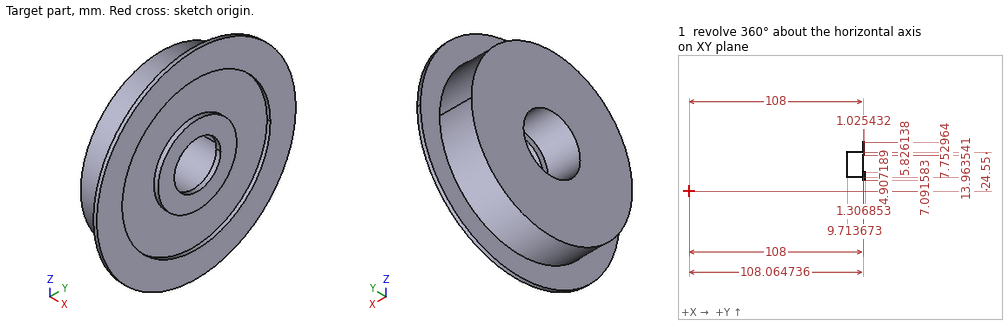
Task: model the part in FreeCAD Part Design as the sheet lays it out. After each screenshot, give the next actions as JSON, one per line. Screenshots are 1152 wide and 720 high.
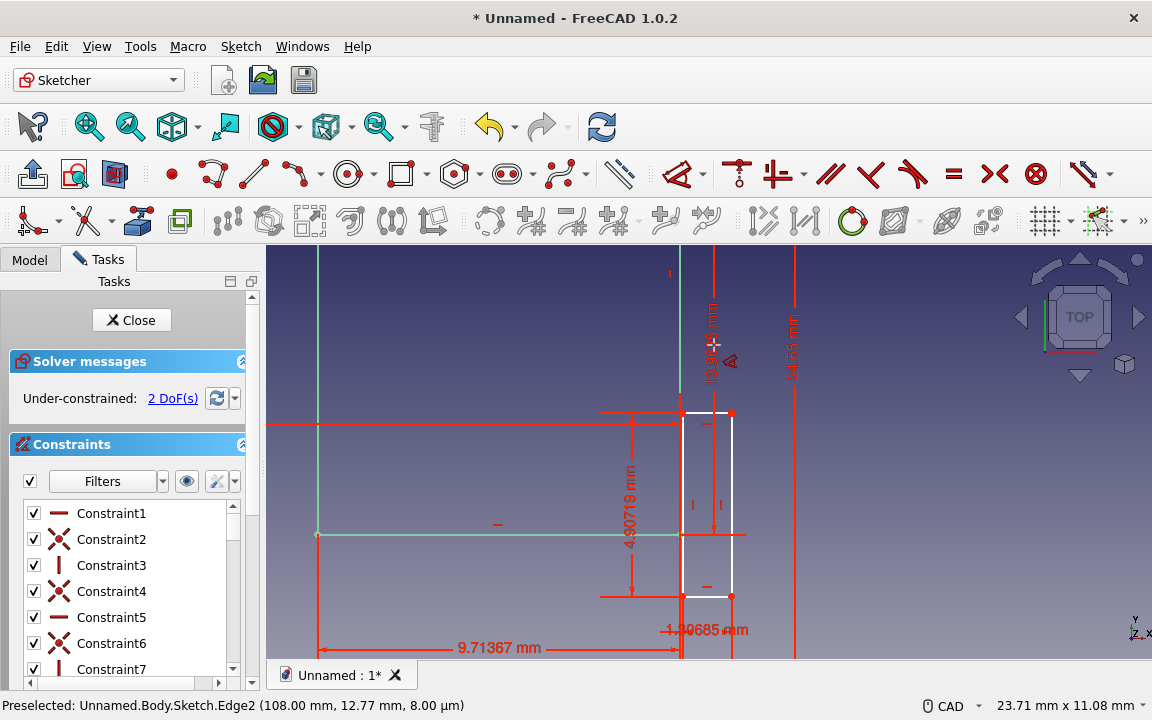
{"action": "left_click", "coordinate": [683, 597]}
{"action": "left_click", "coordinate": [741, 606]}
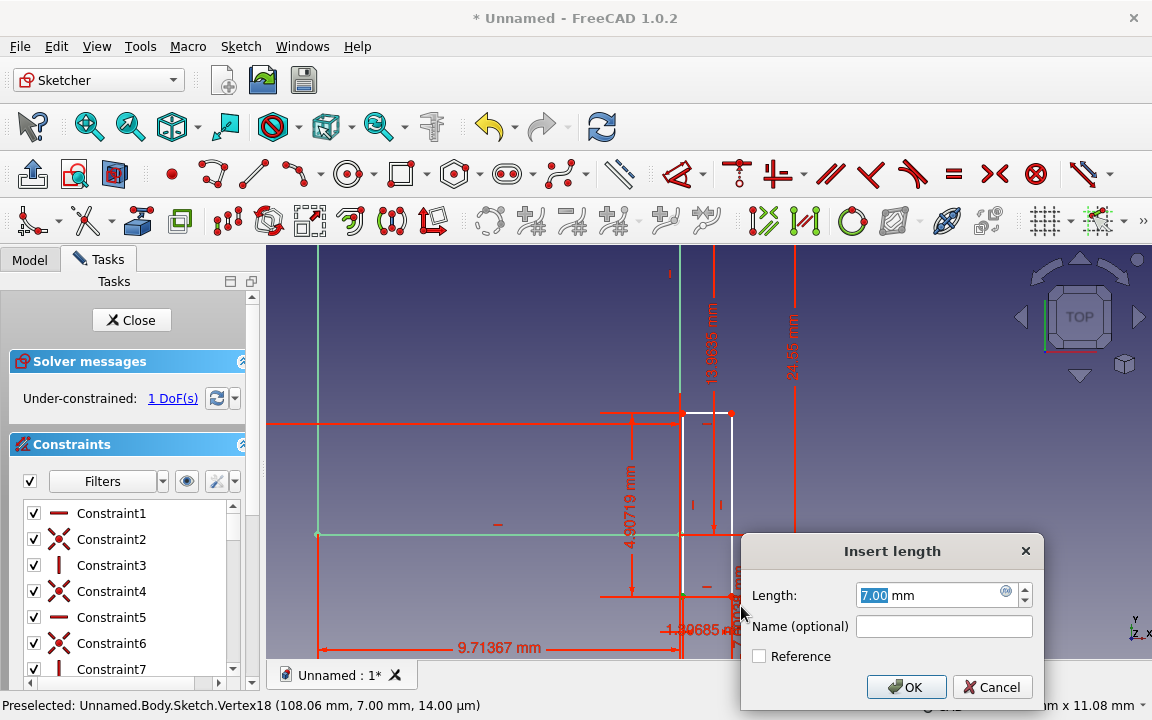
{"action": "type", "text": "7.091583"}
{"action": "key", "text": "Return"}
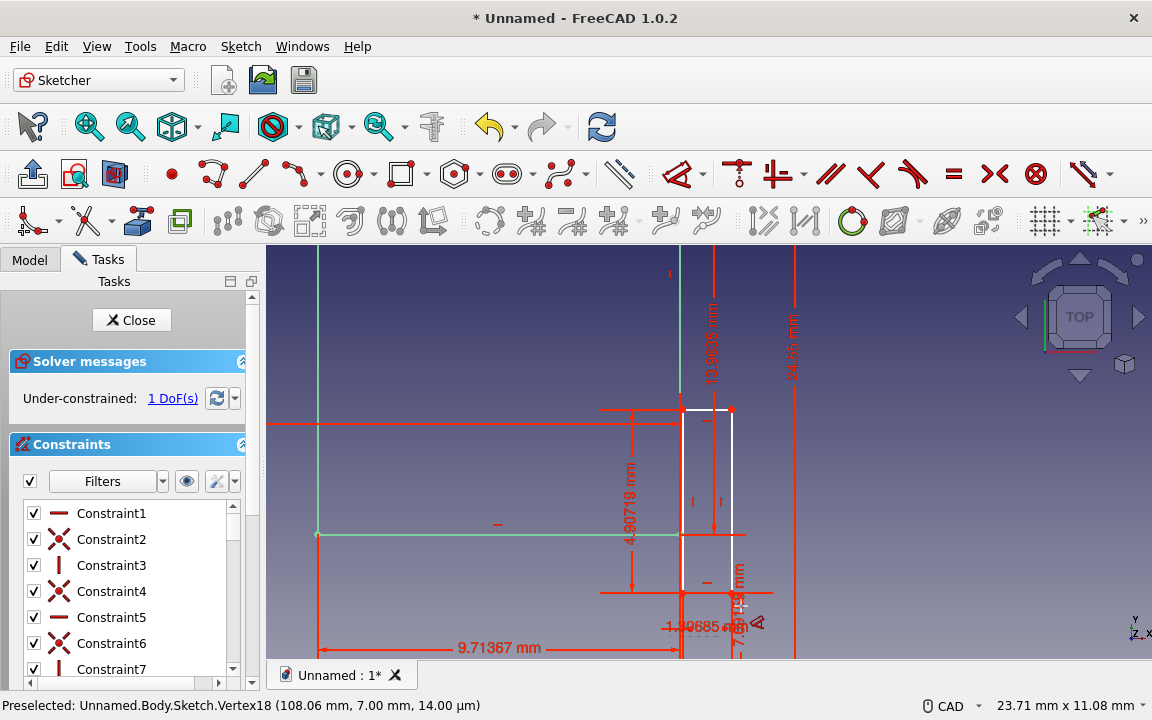
{"action": "left_click", "coordinate": [683, 410]}
{"action": "left_click", "coordinate": [488, 376]}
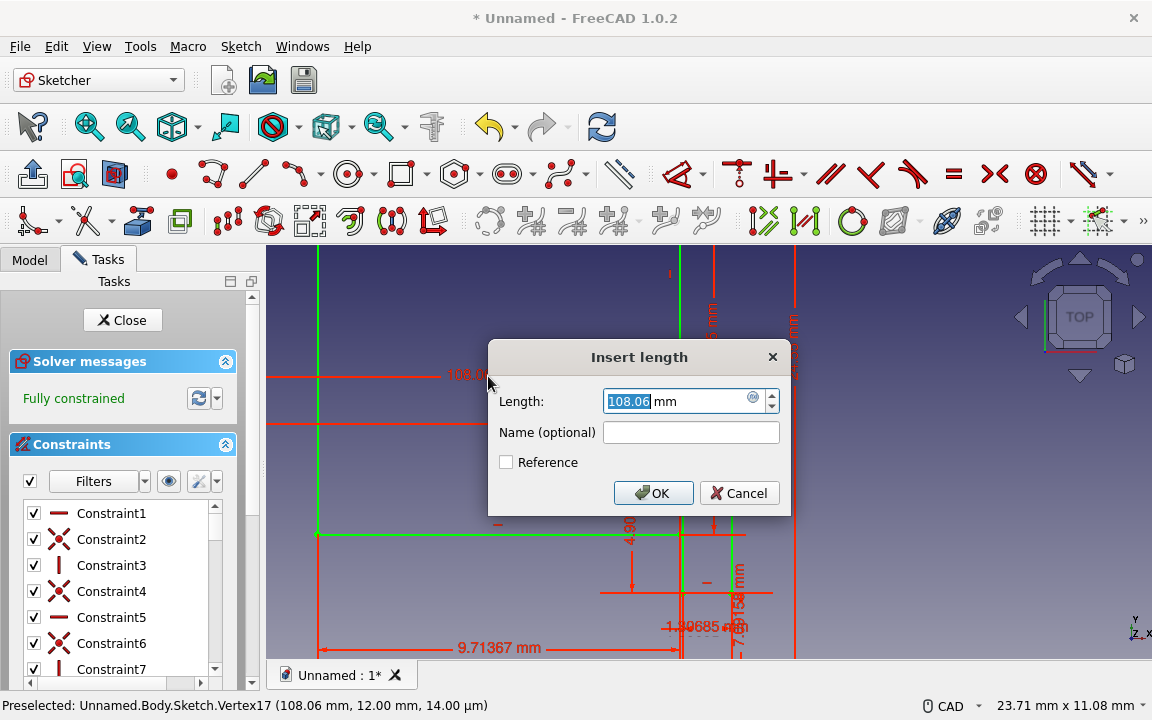
{"action": "type", "text": "108.064736"}
{"action": "key", "text": "Return"}
{"action": "key", "text": "Escape"}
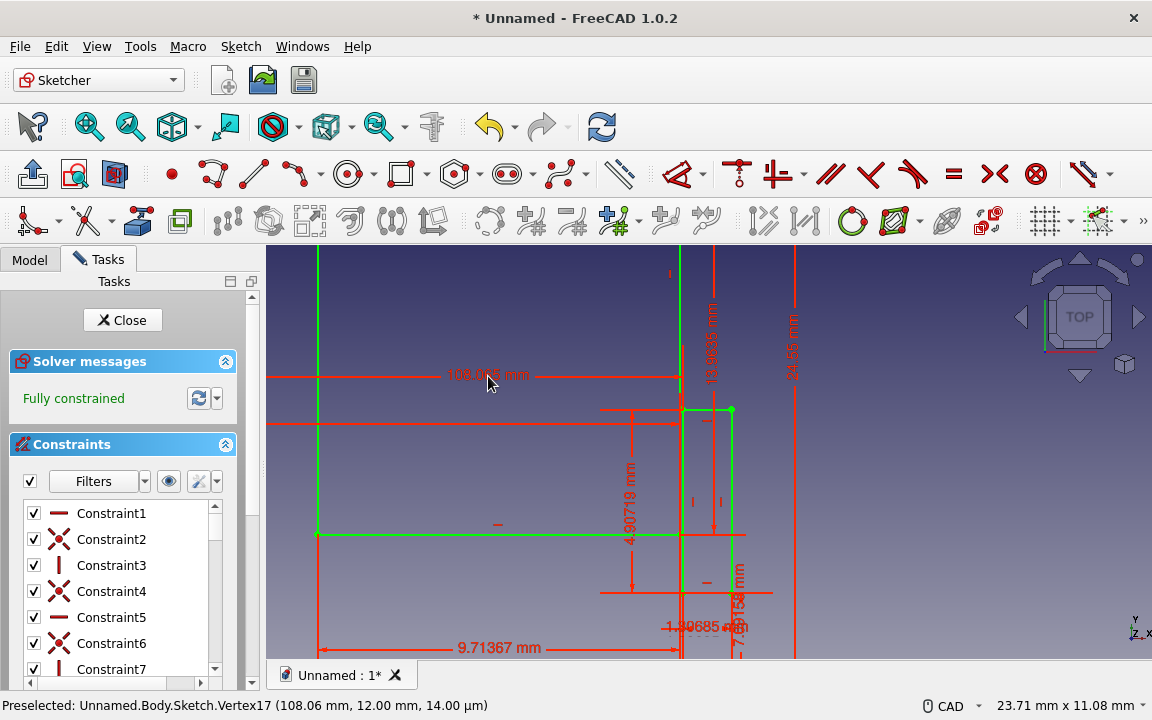
{"action": "left_click", "coordinate": [123, 320]}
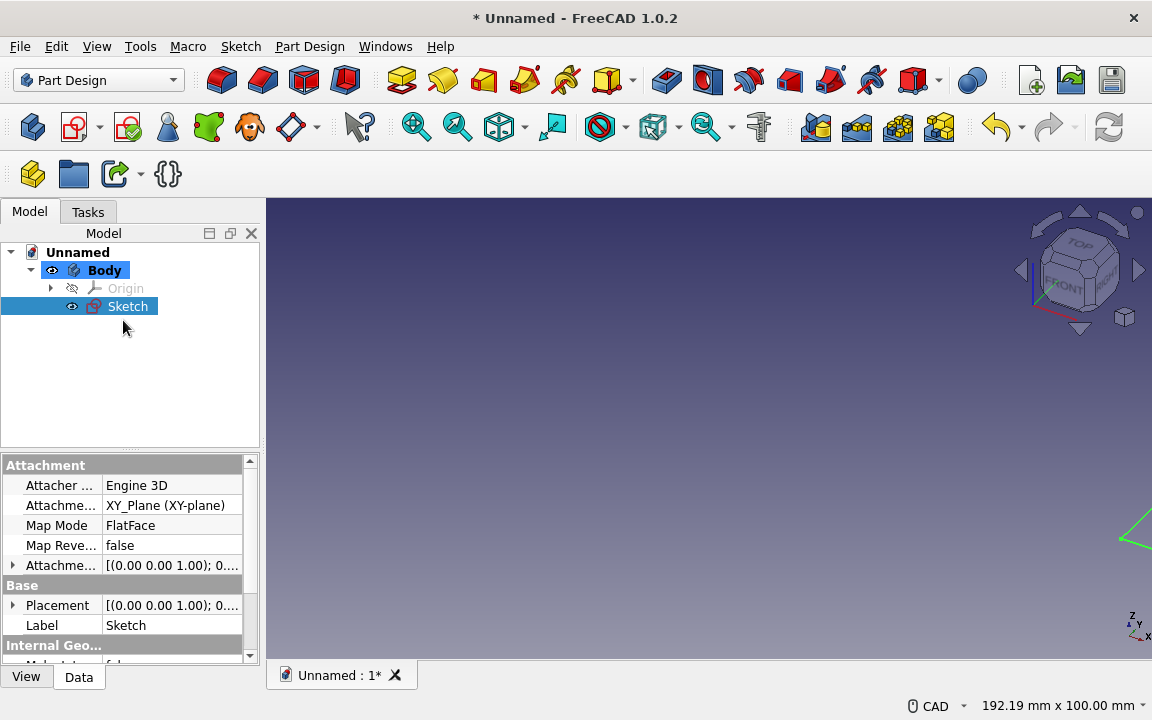
{"action": "left_click", "coordinate": [443, 80]}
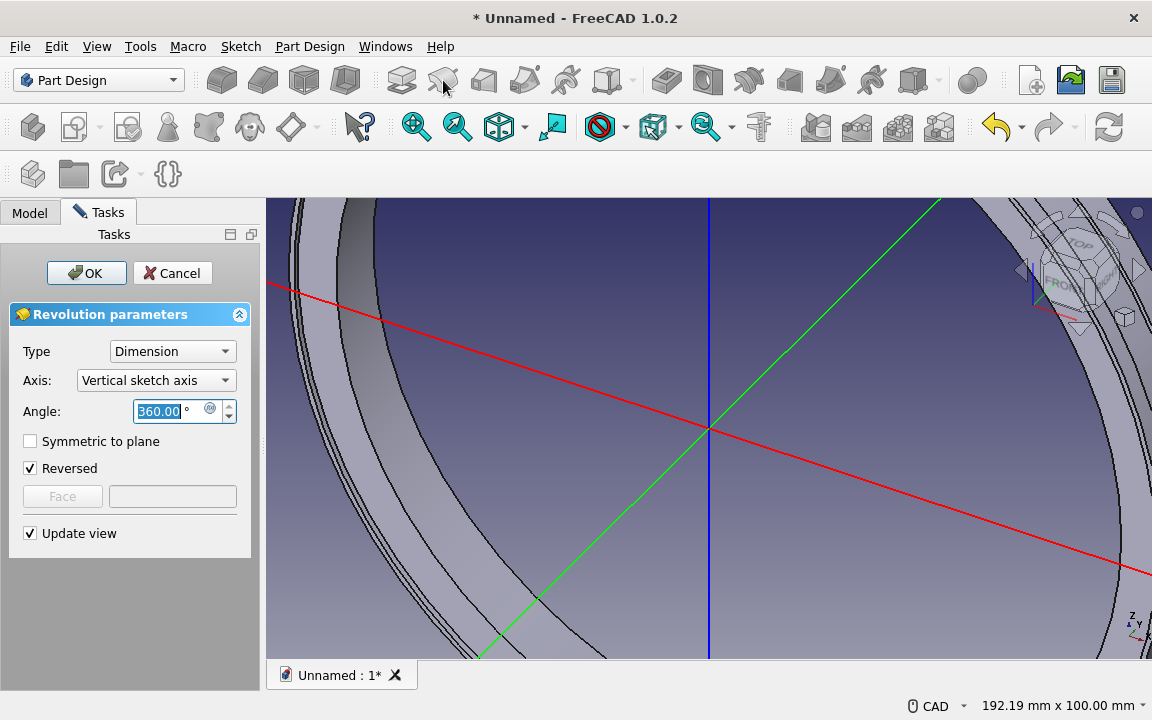
{"action": "left_click", "coordinate": [157, 380]}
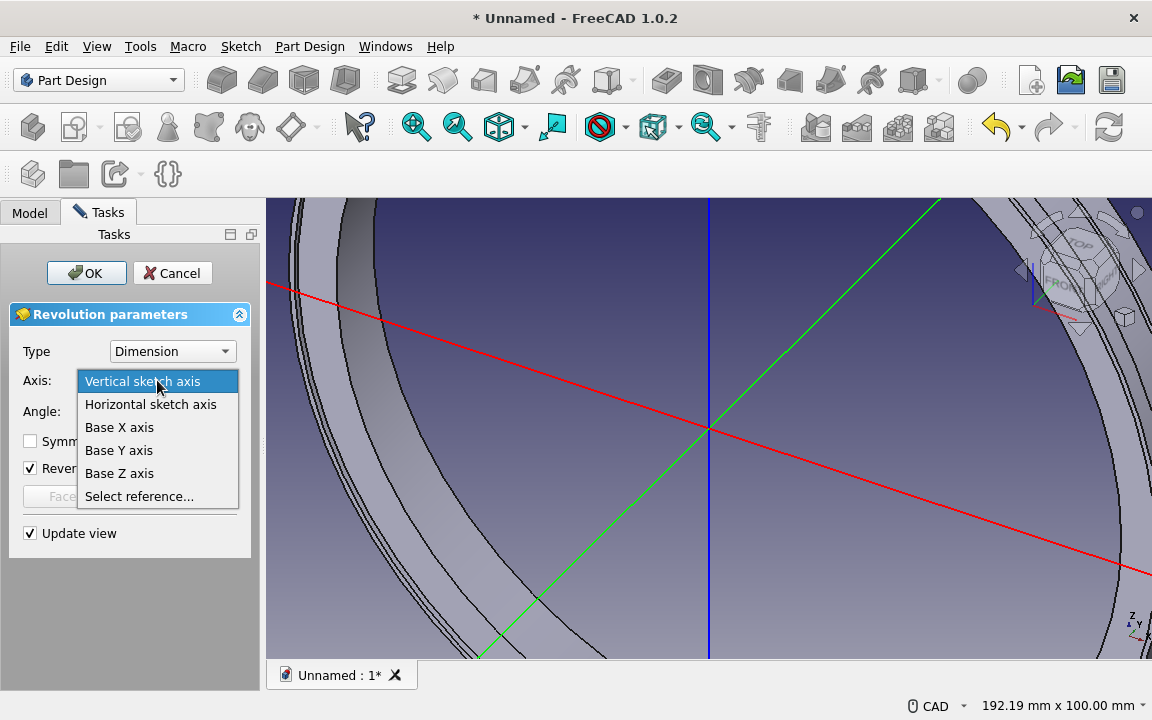
{"action": "left_click", "coordinate": [156, 404]}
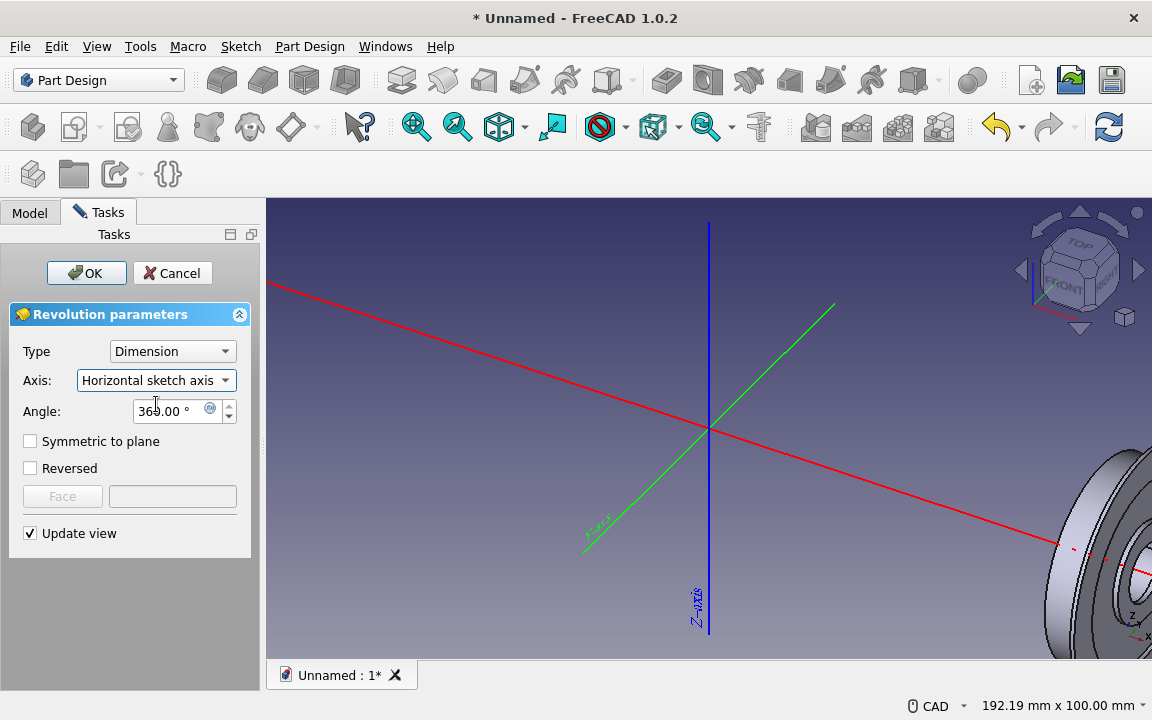
{"action": "left_click", "coordinate": [87, 273]}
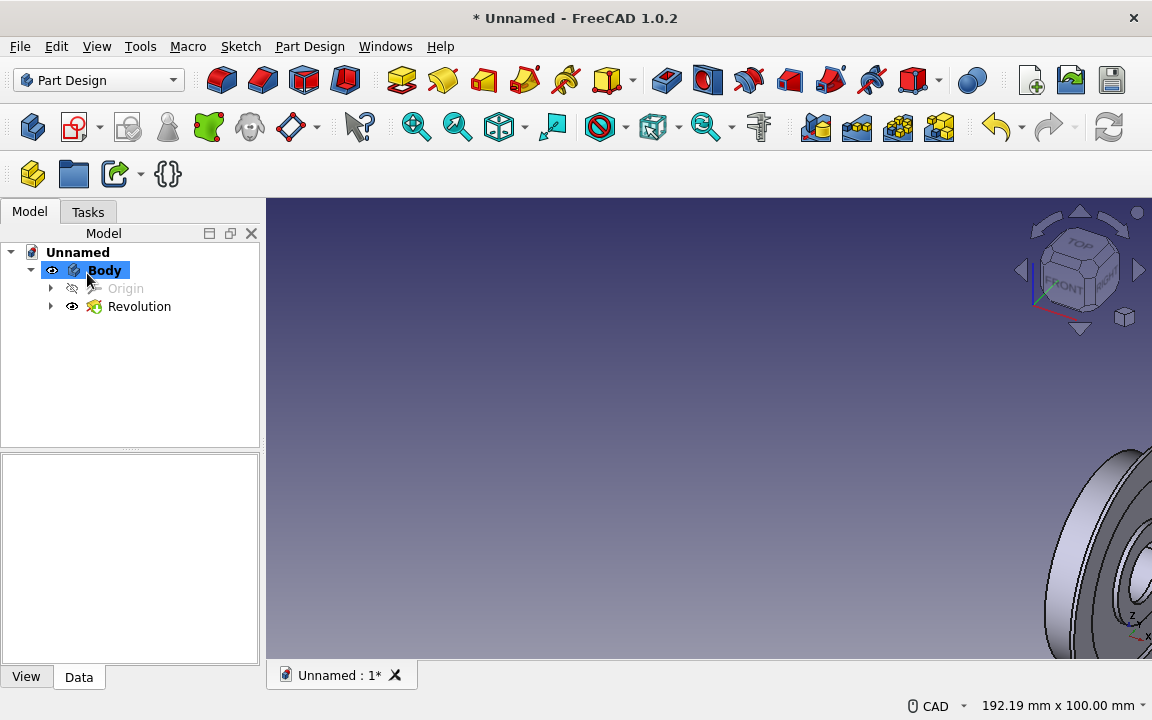
{"action": "key", "text": "0"}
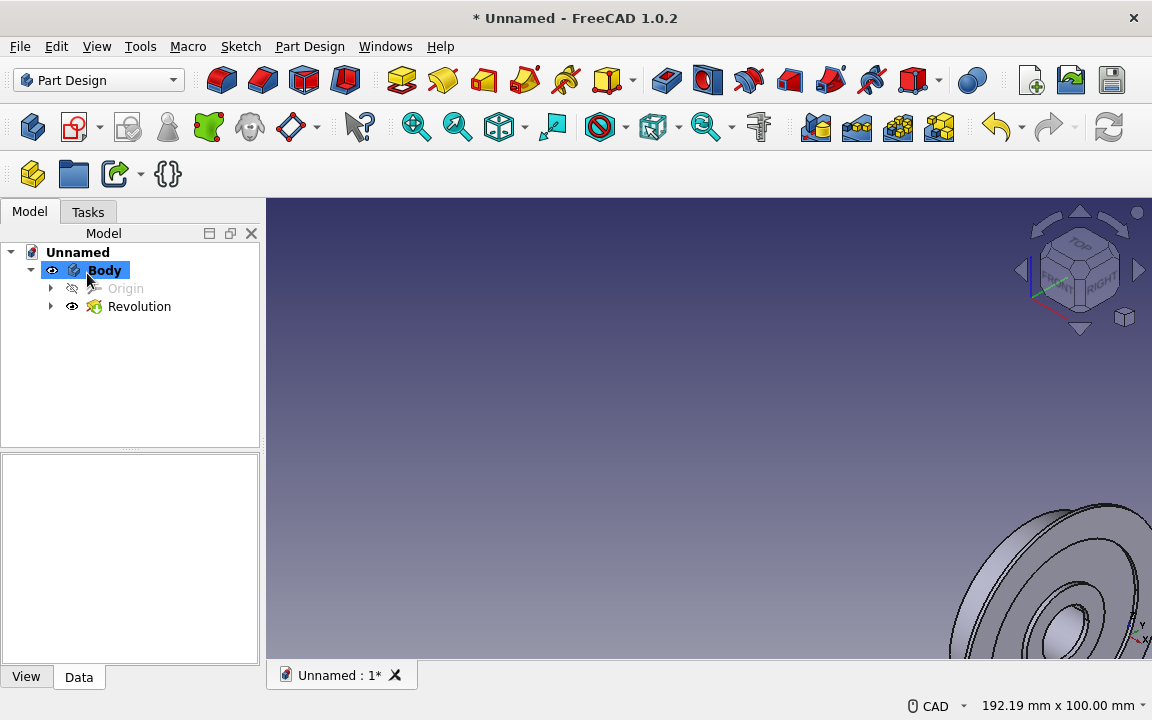
{"action": "left_click", "coordinate": [417, 128]}